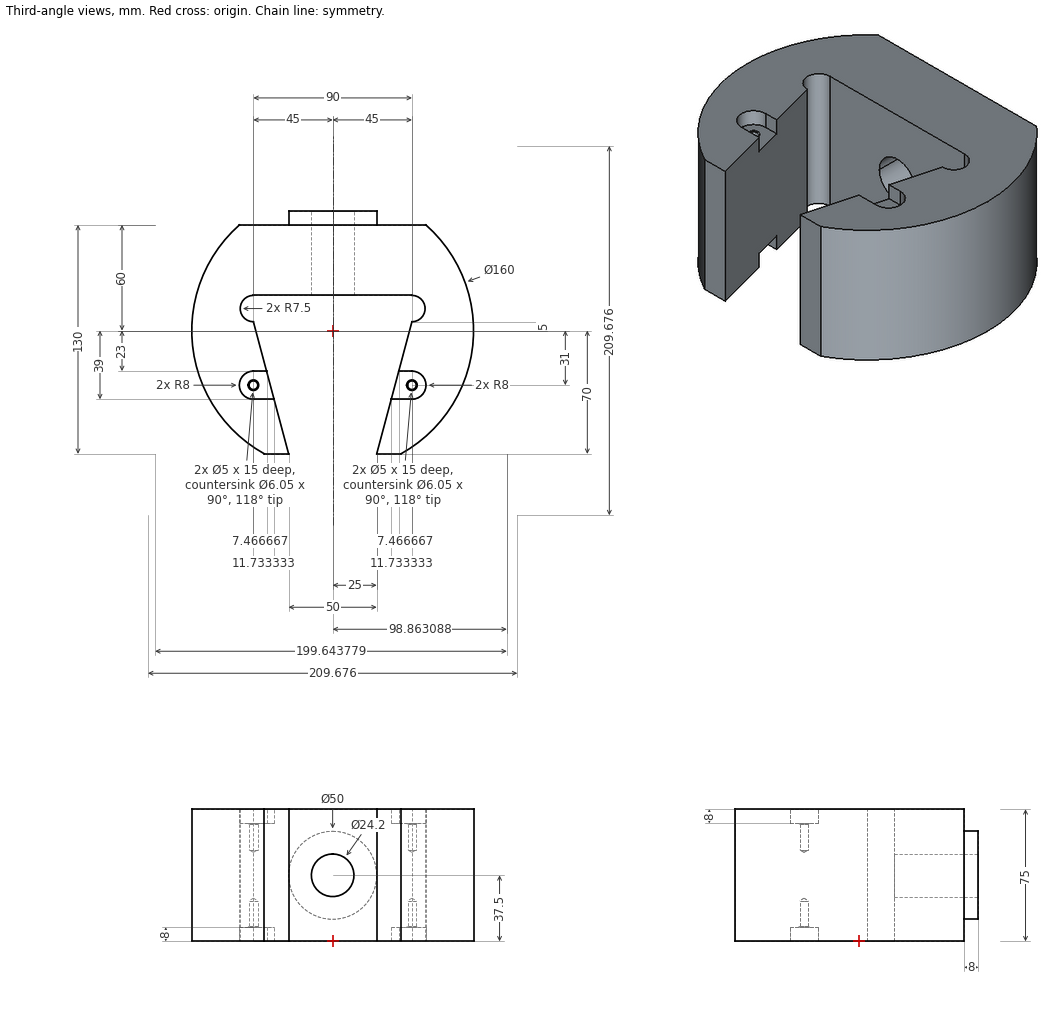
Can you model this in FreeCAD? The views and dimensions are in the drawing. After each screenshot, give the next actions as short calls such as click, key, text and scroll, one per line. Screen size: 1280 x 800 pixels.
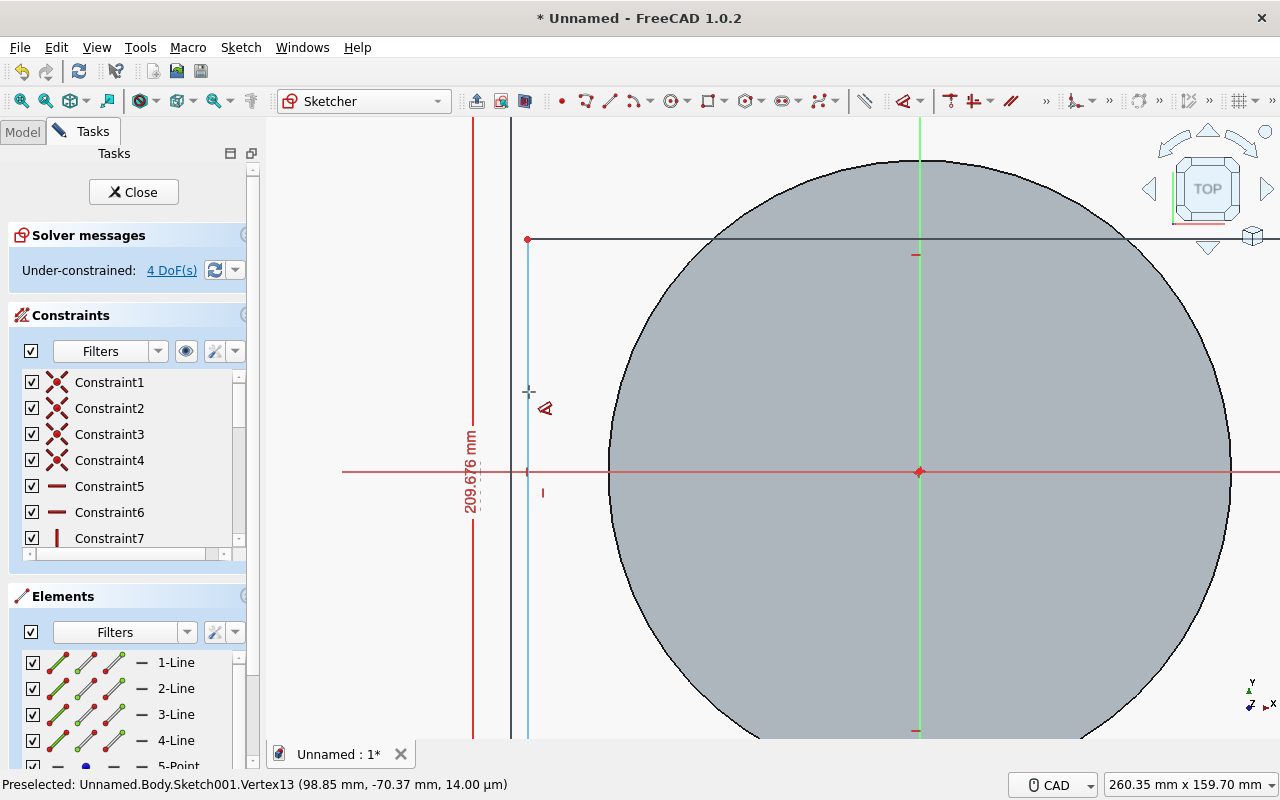
click(528, 391)
click(494, 367)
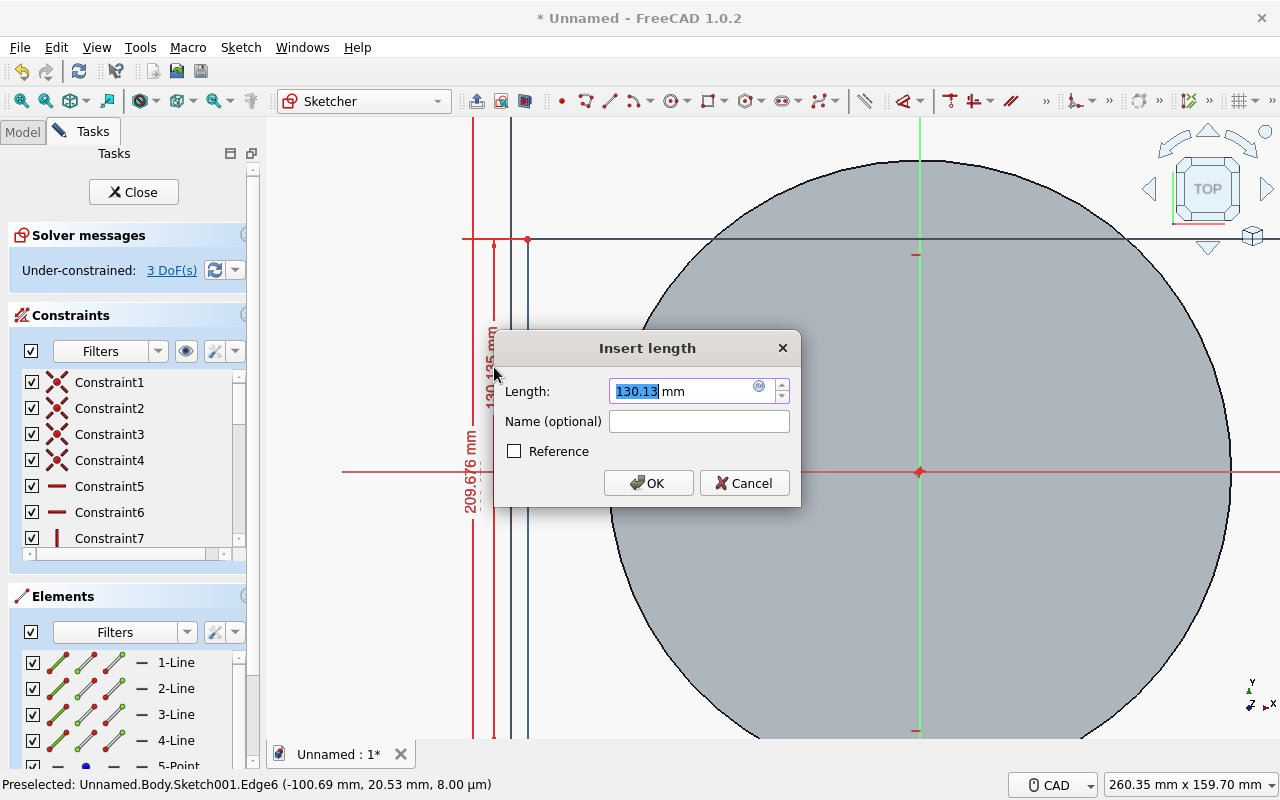
text(130)
key(Return)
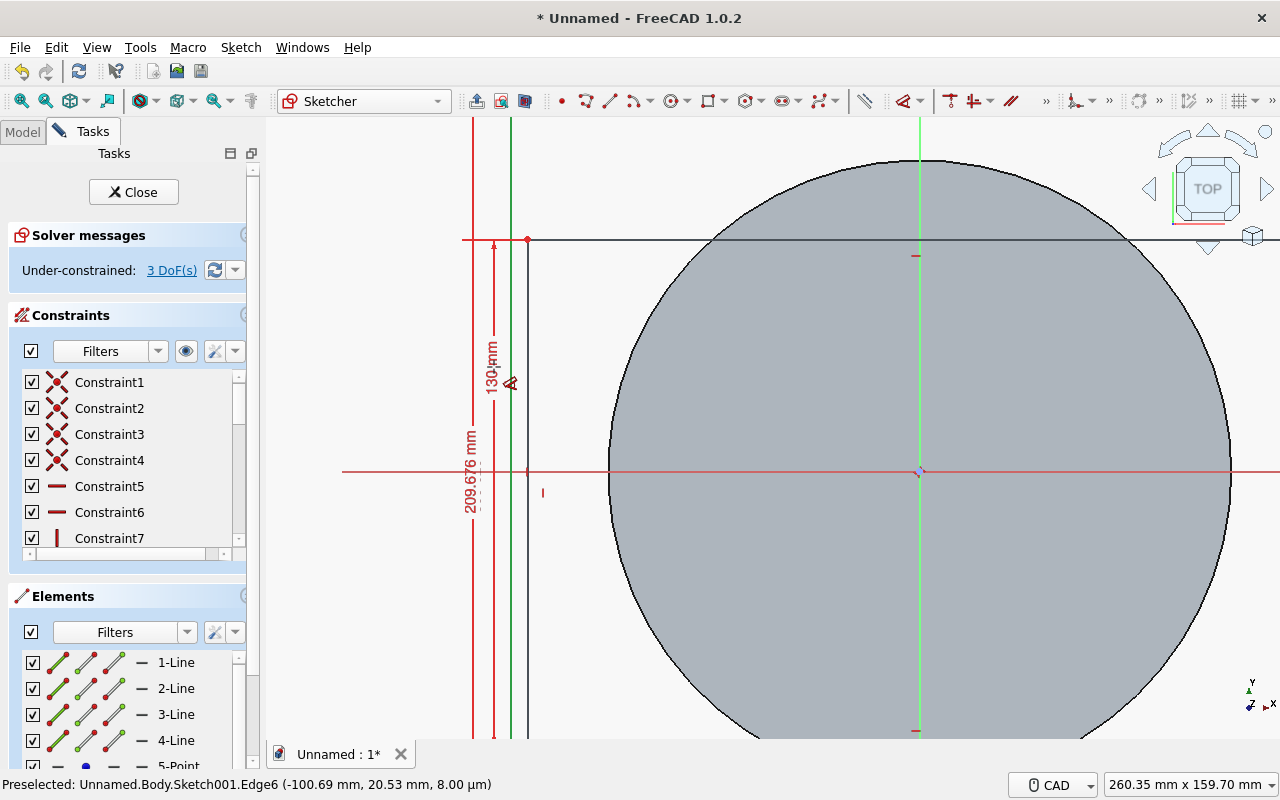
click(528, 240)
click(494, 302)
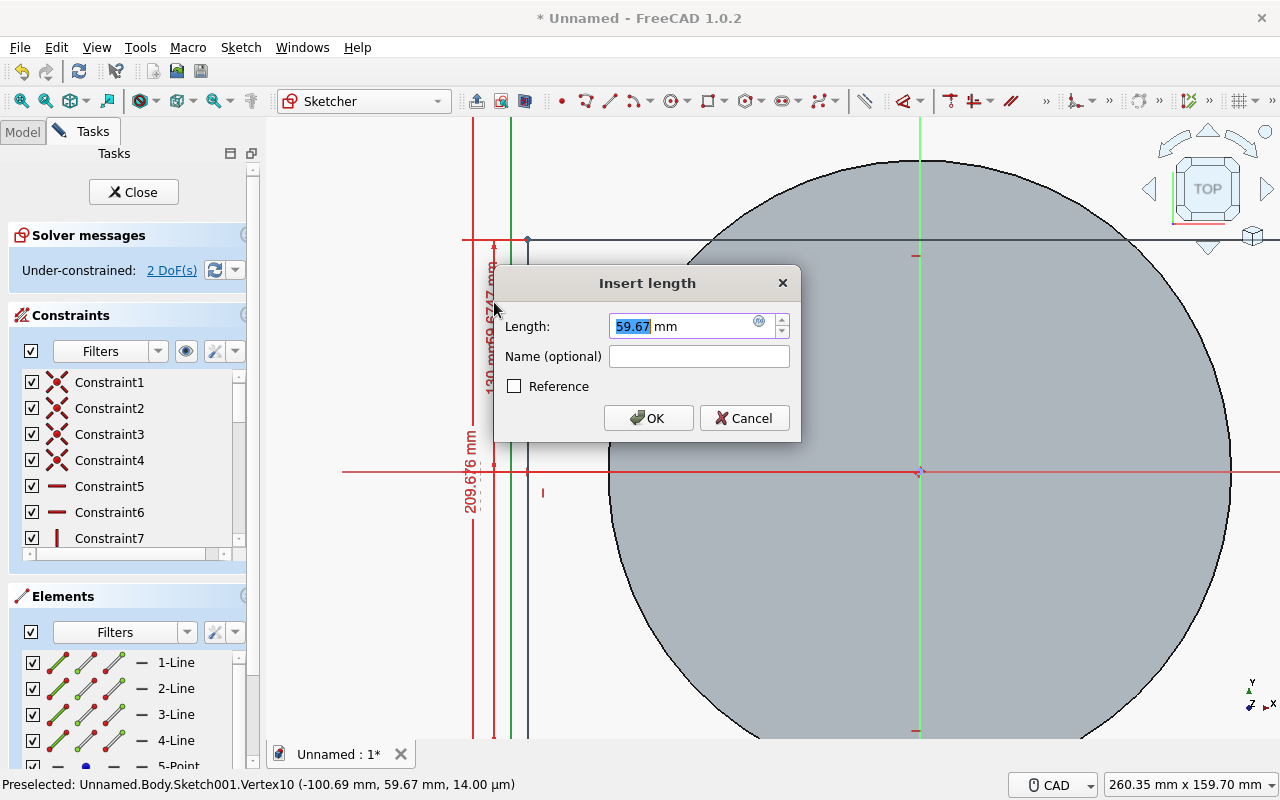
text(60)
key(Return)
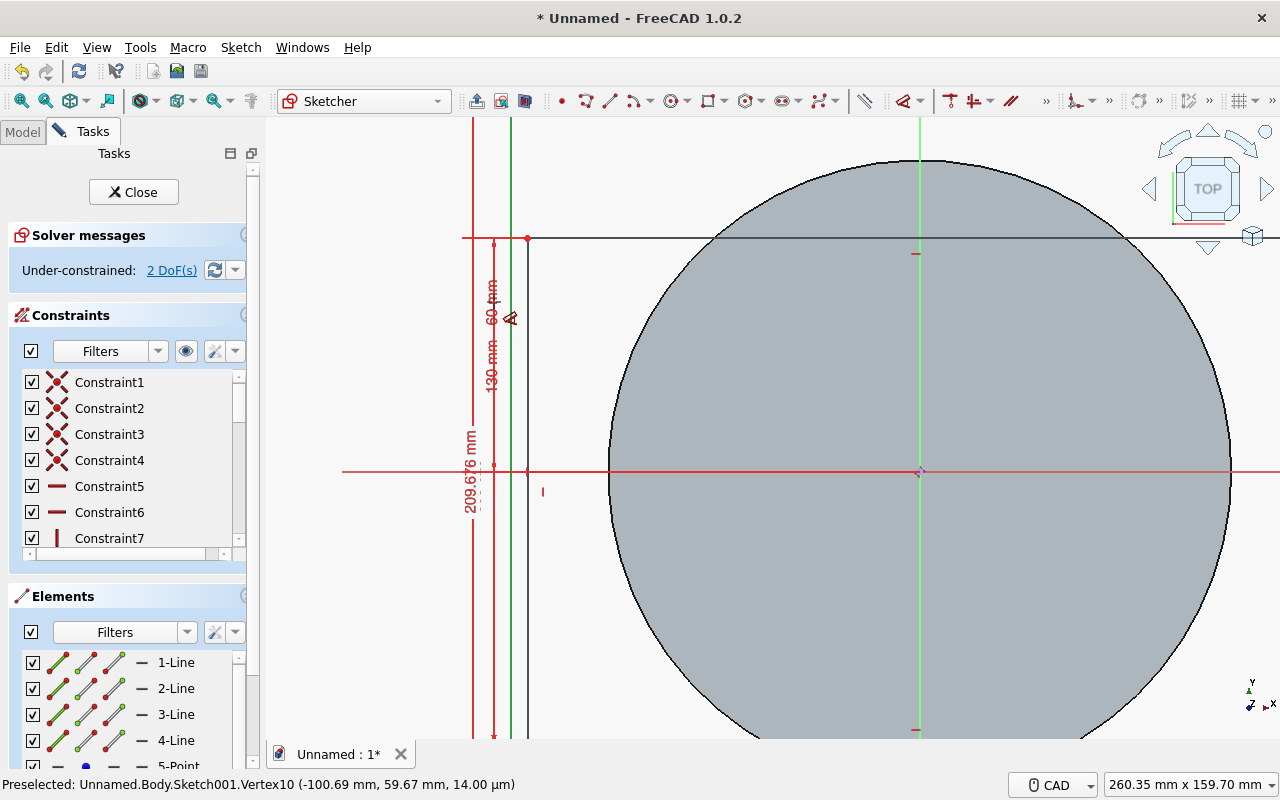
scroll(529, 392, down, 4)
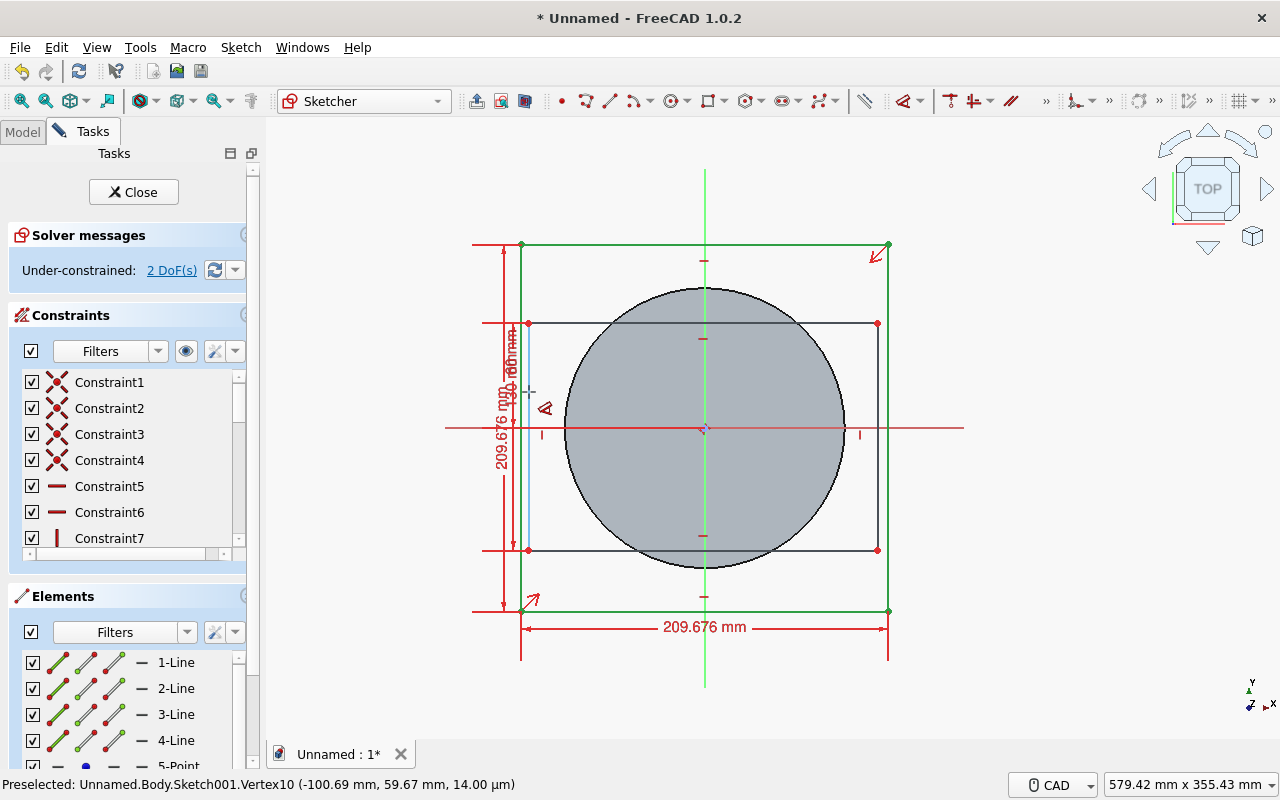
click(633, 551)
click(623, 585)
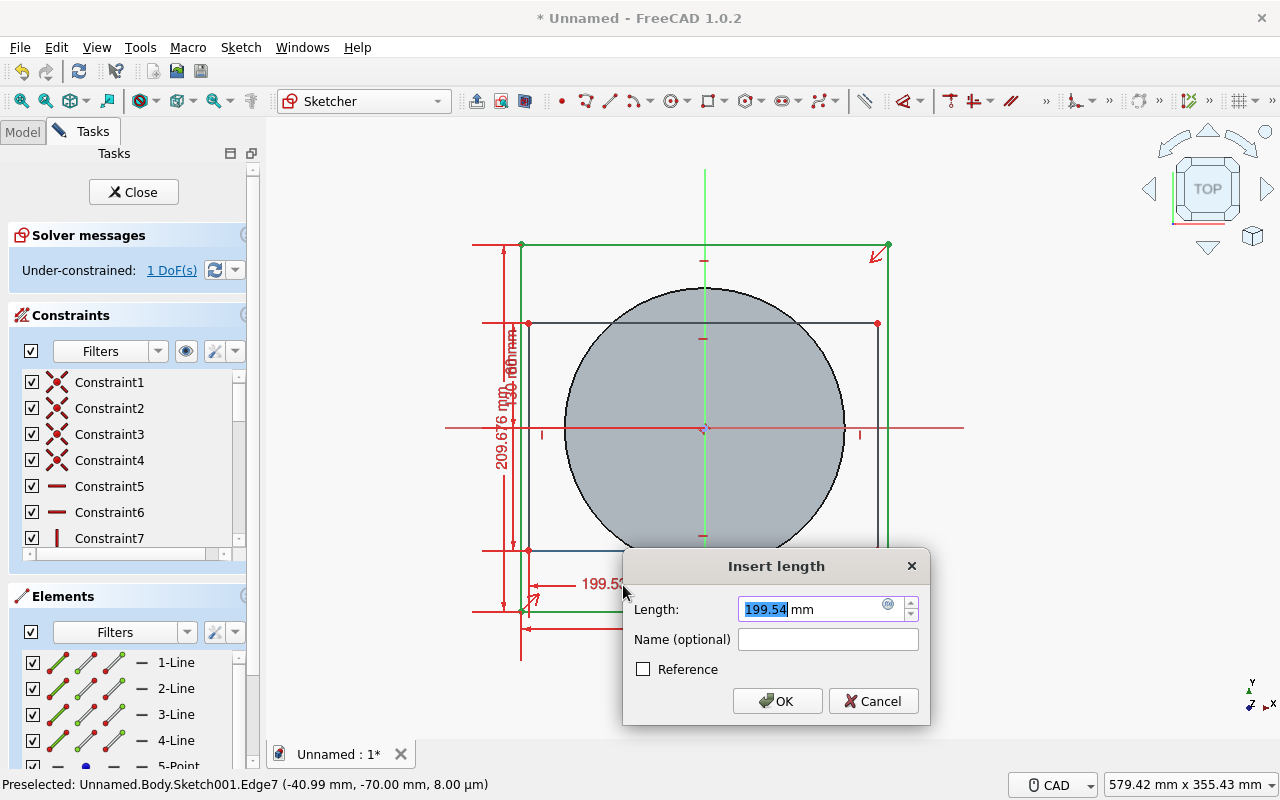
text(199.643779)
key(Return)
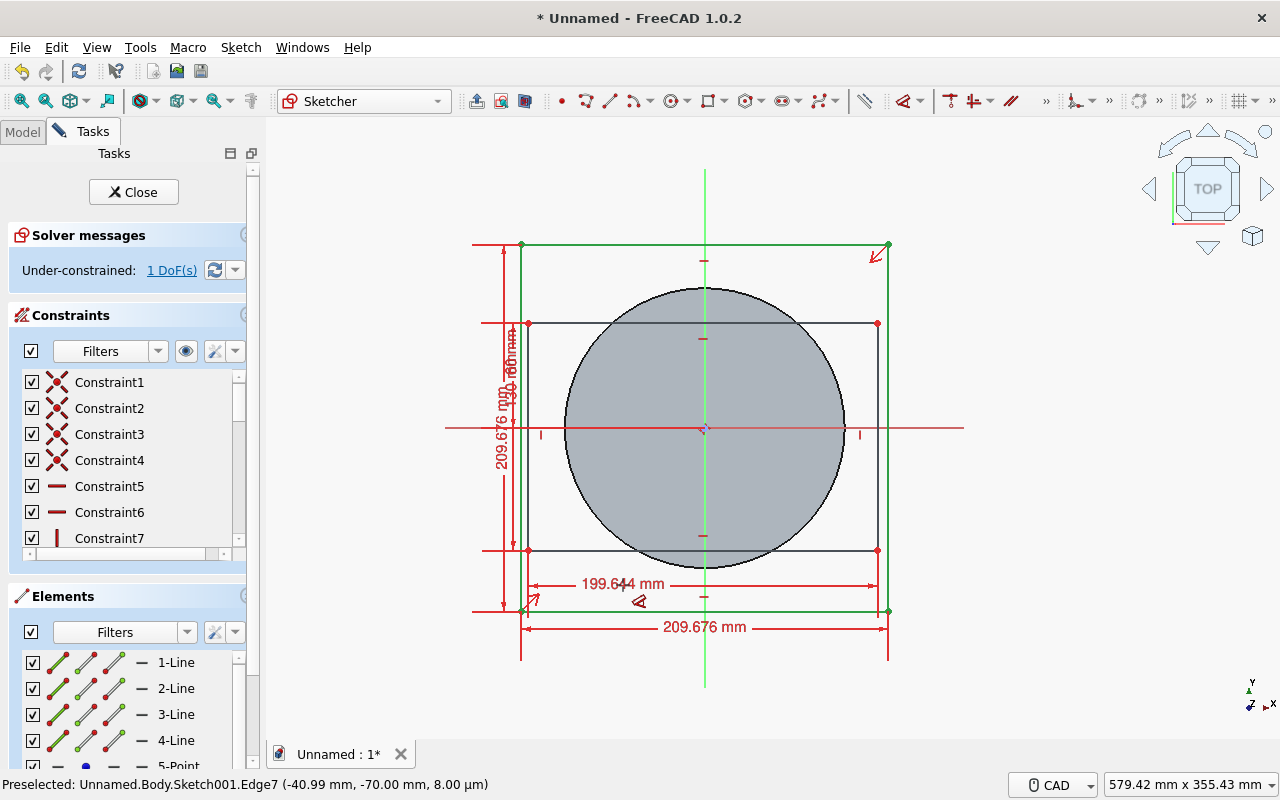
click(878, 551)
click(791, 585)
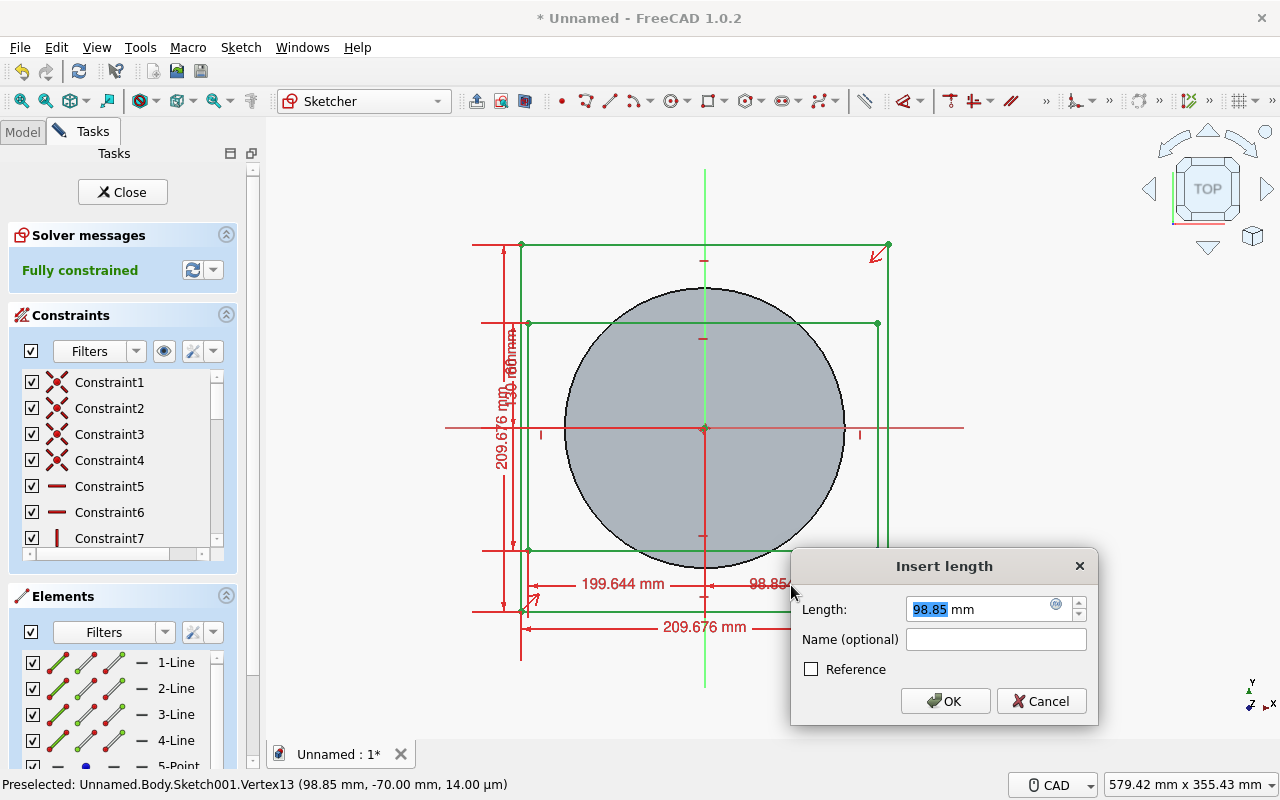
text(98.863088)
key(Return)
key(Escape)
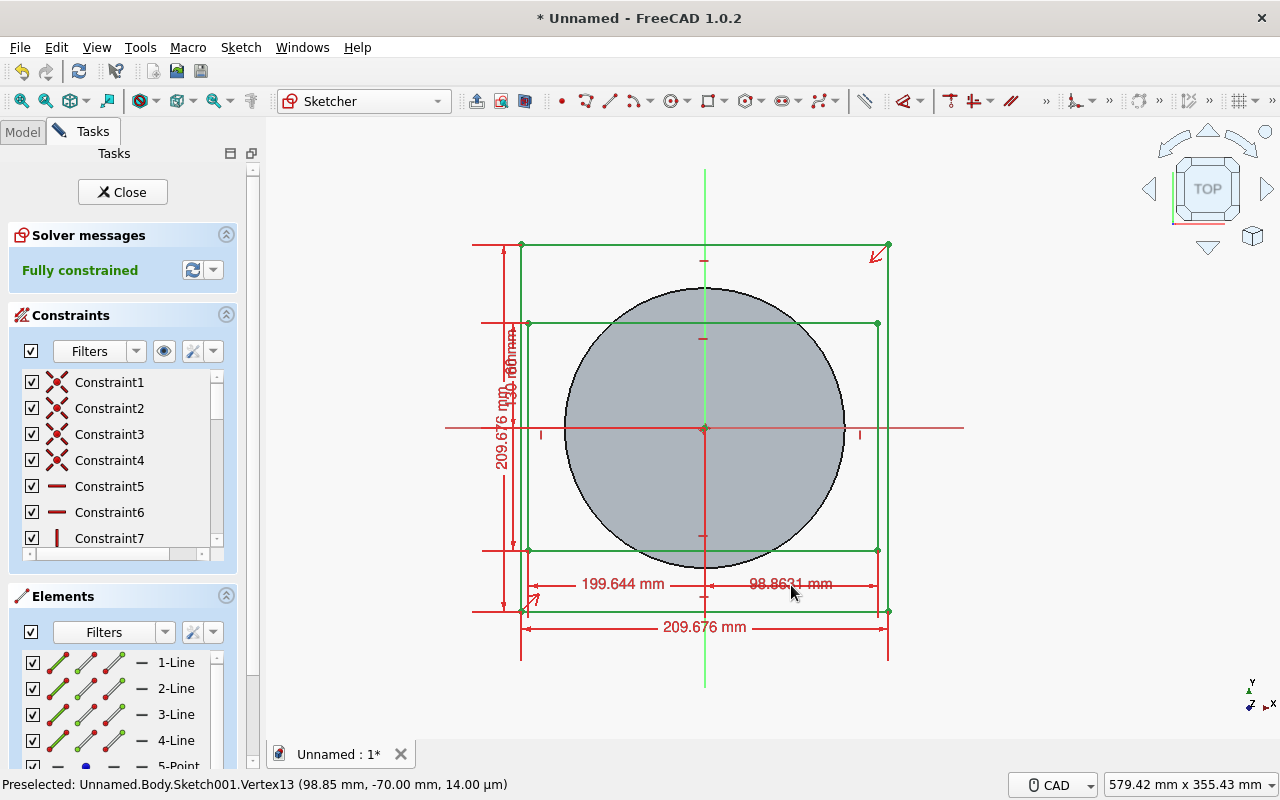
click(123, 192)